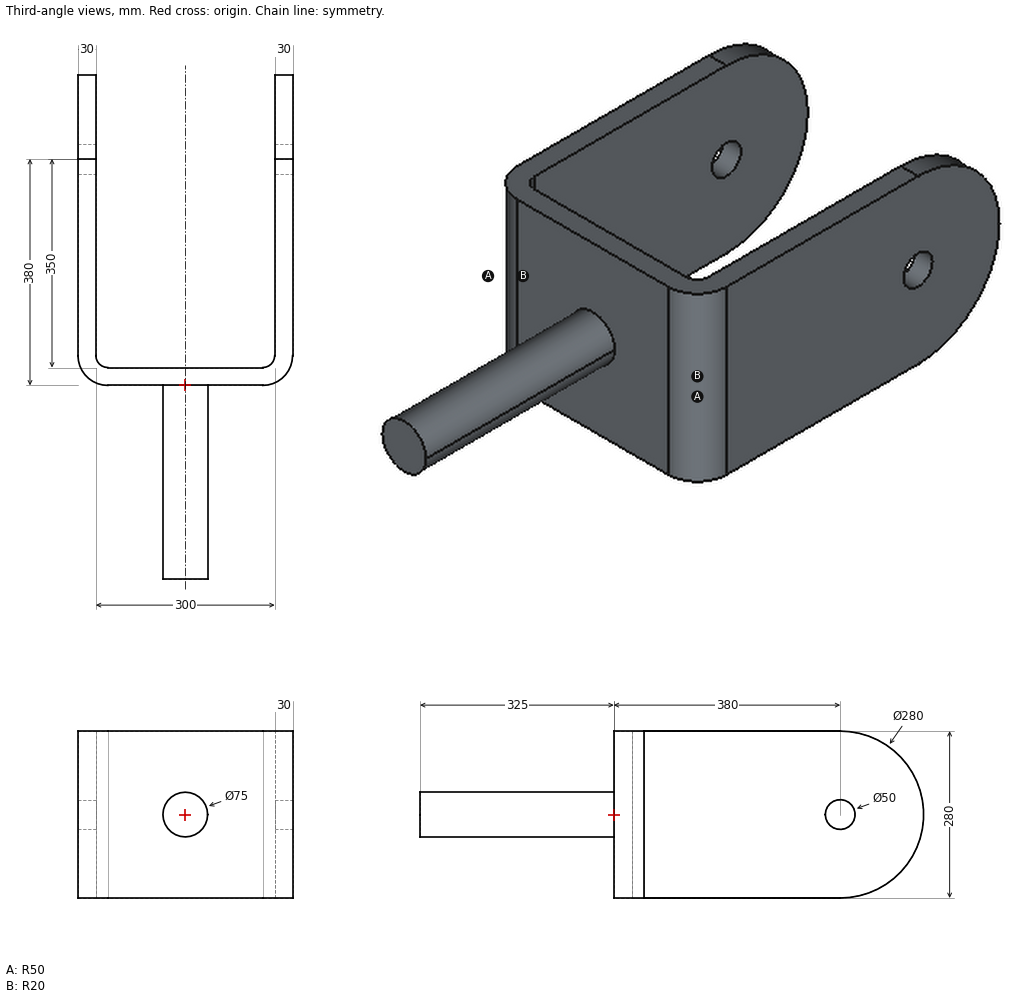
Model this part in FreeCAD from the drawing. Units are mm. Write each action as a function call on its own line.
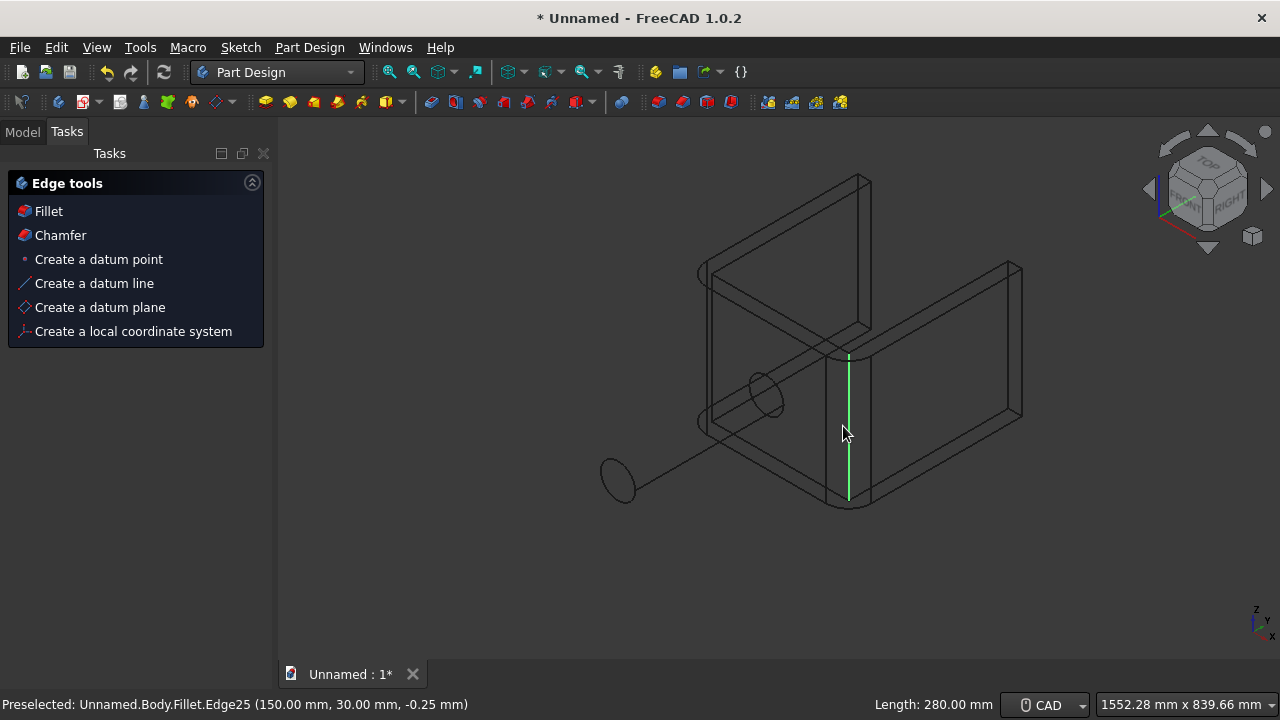
key(2)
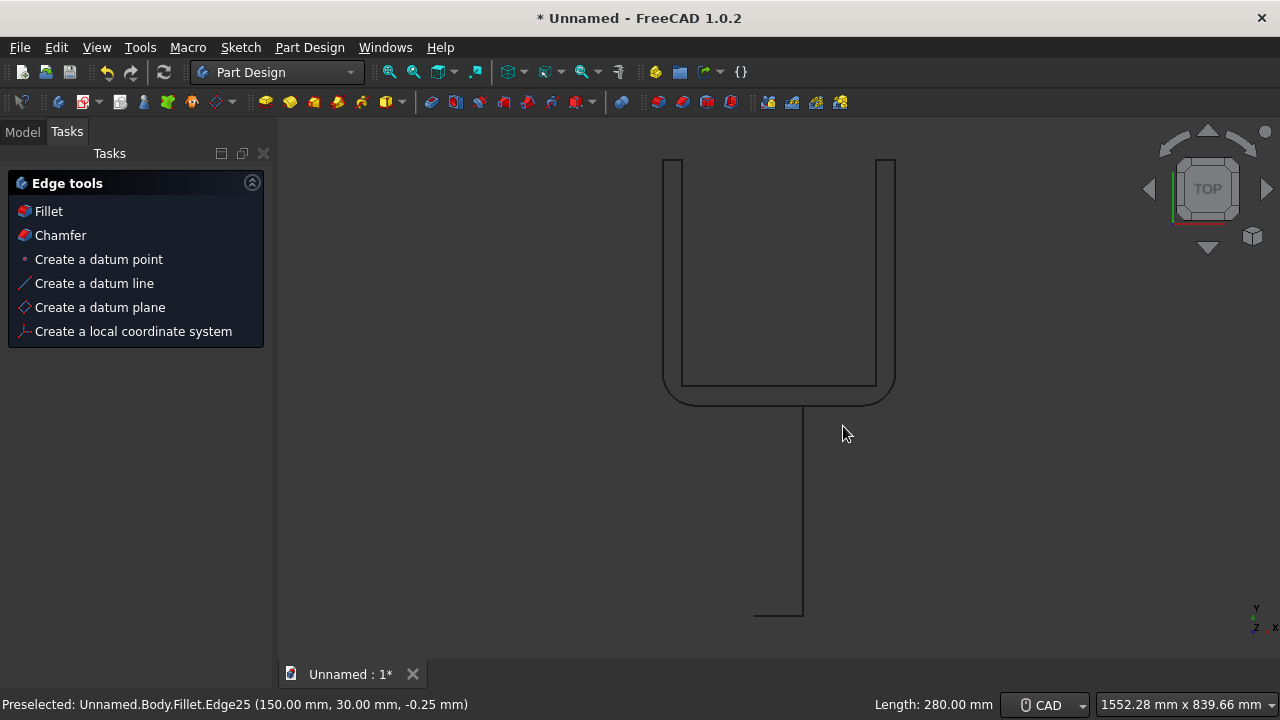
key(1)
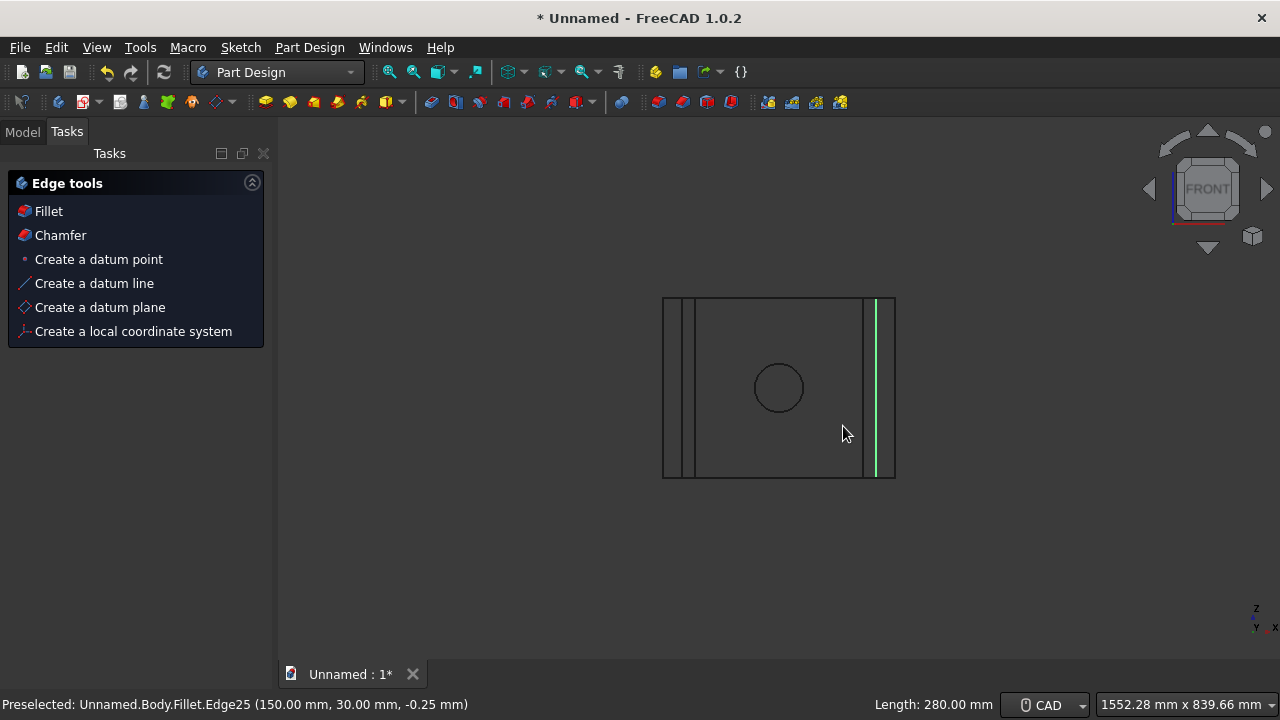
click(390, 72)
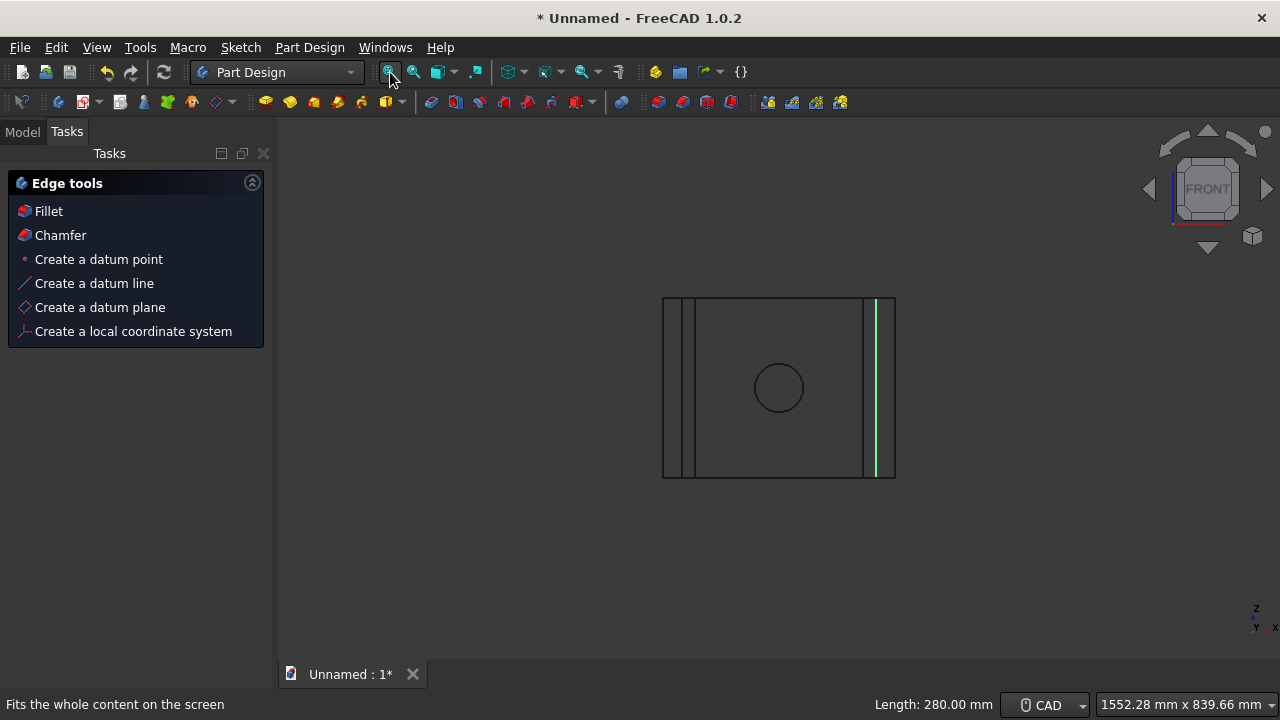
click(682, 387, ctrl)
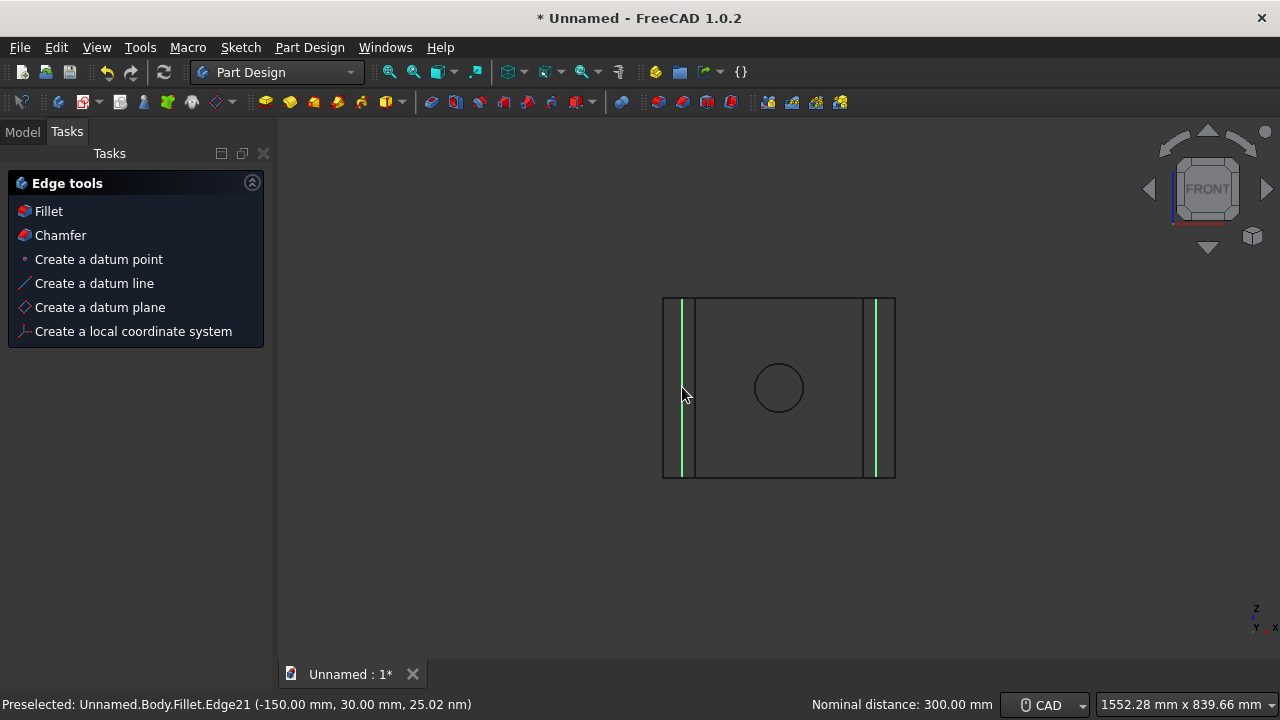
key(v)
key(1)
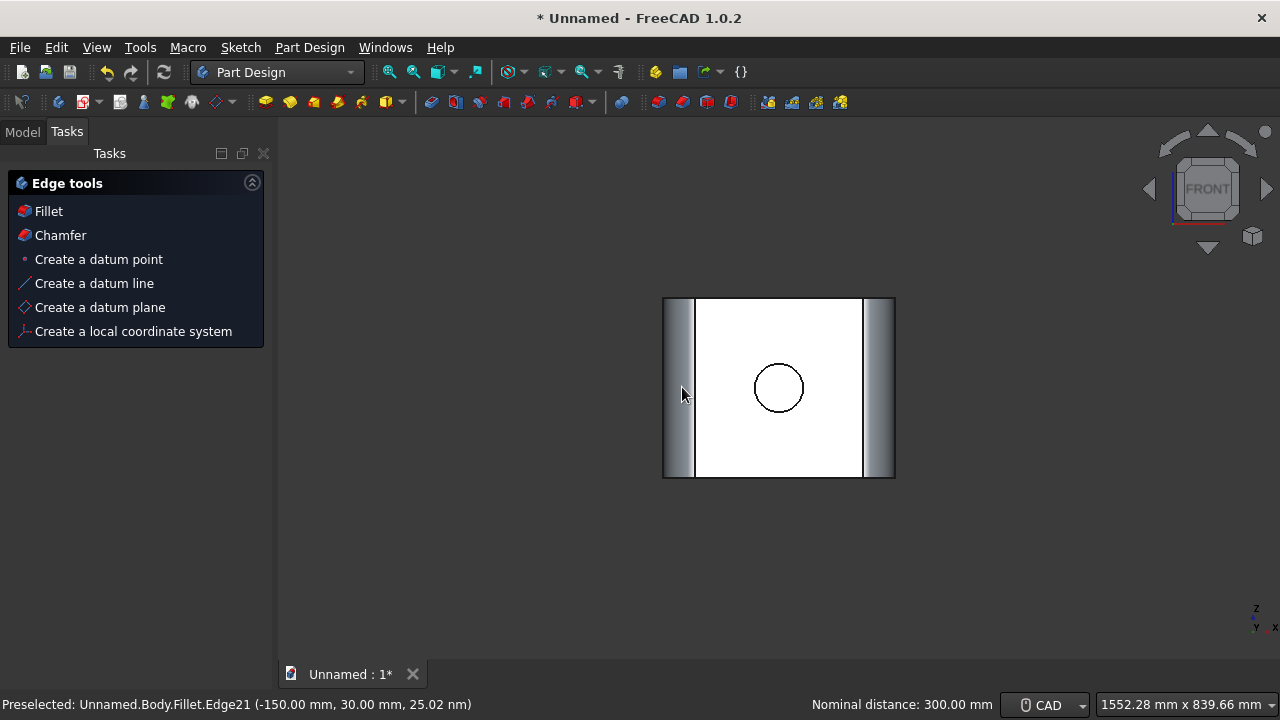
click(660, 102)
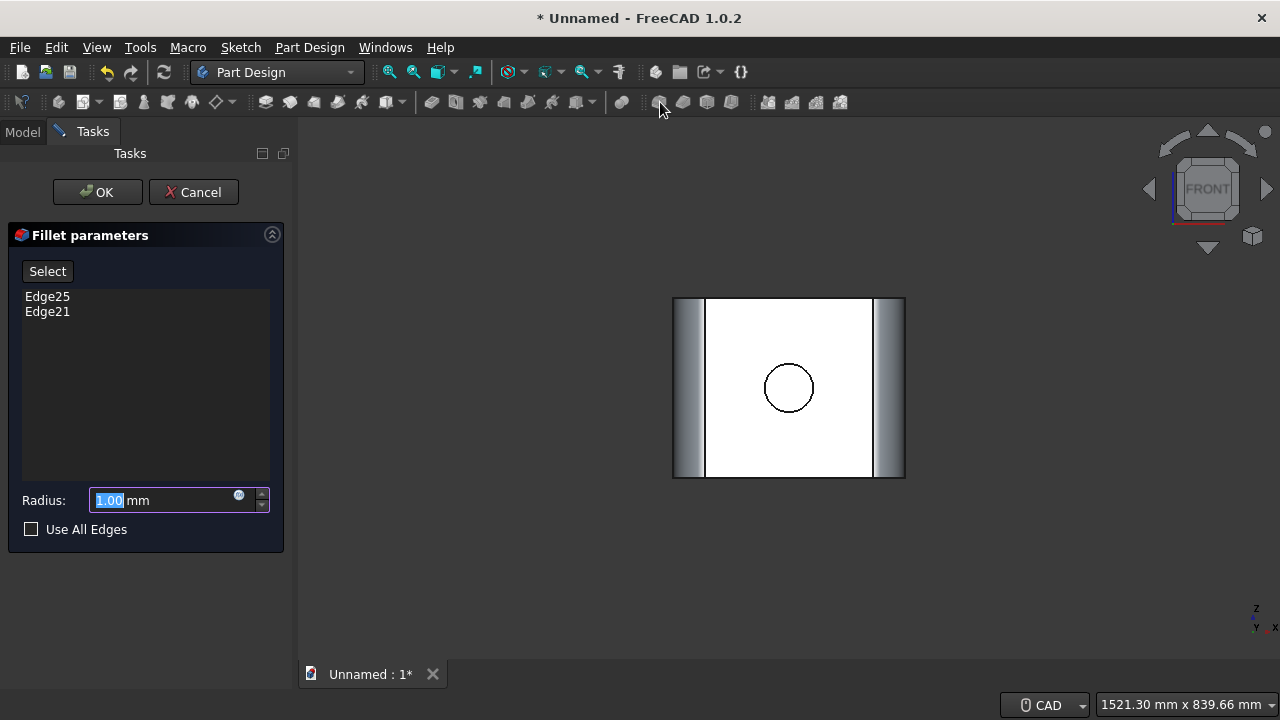
text(20)
key(Tab)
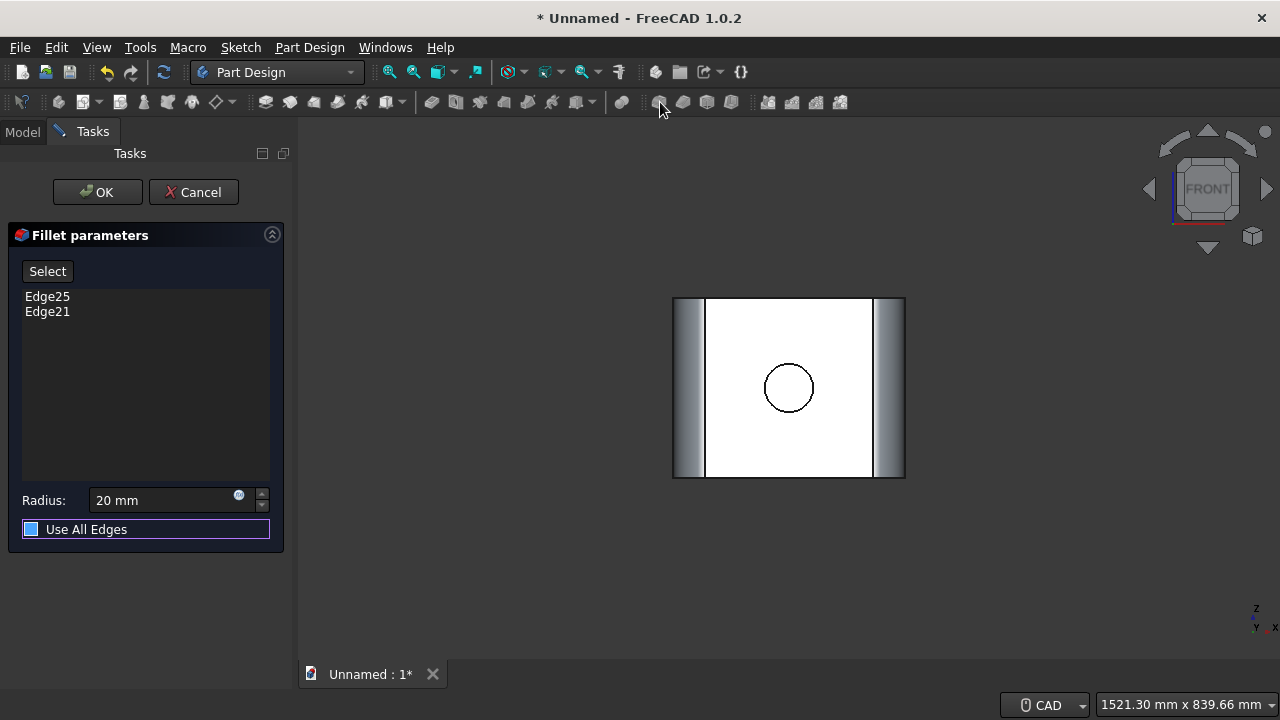
click(98, 192)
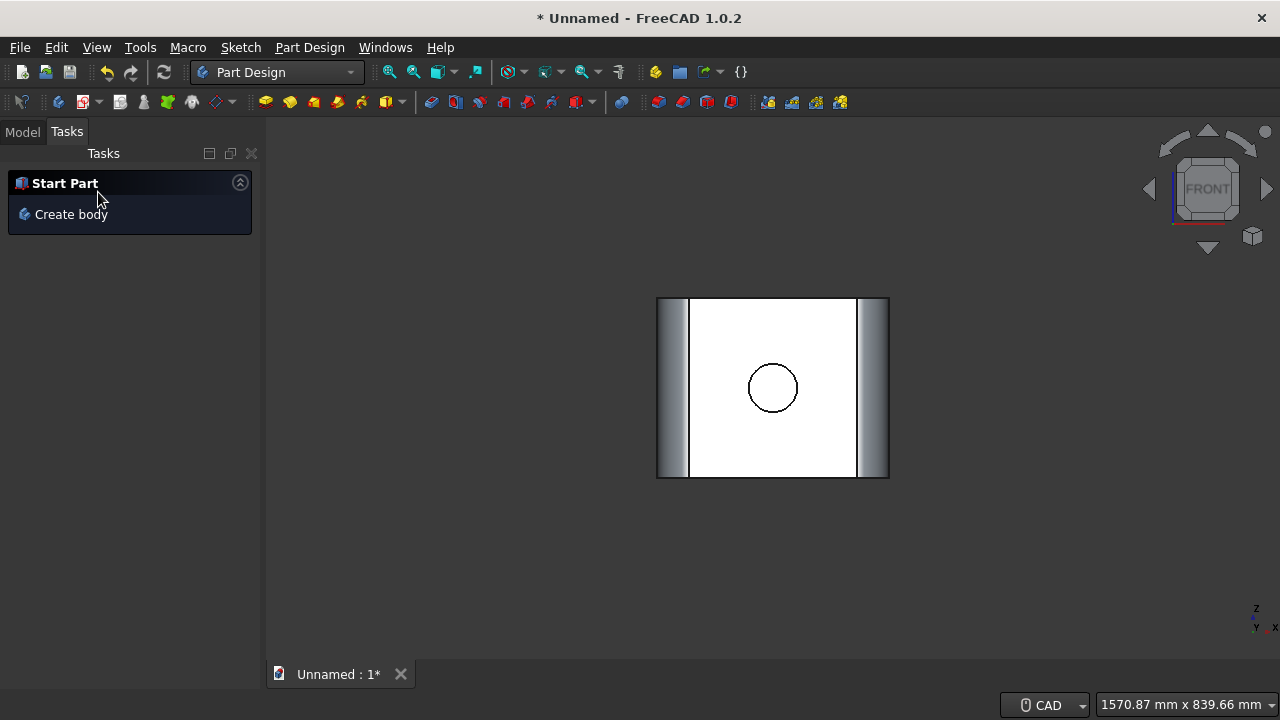
click(390, 72)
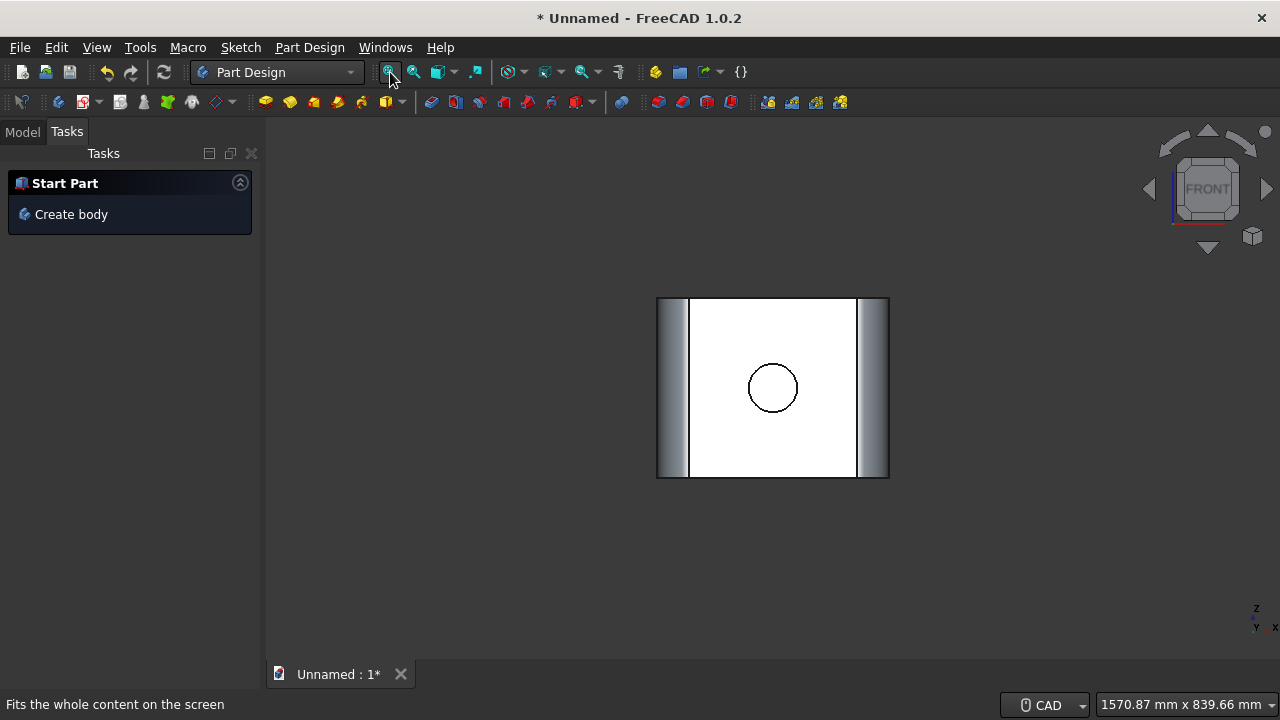
key(0)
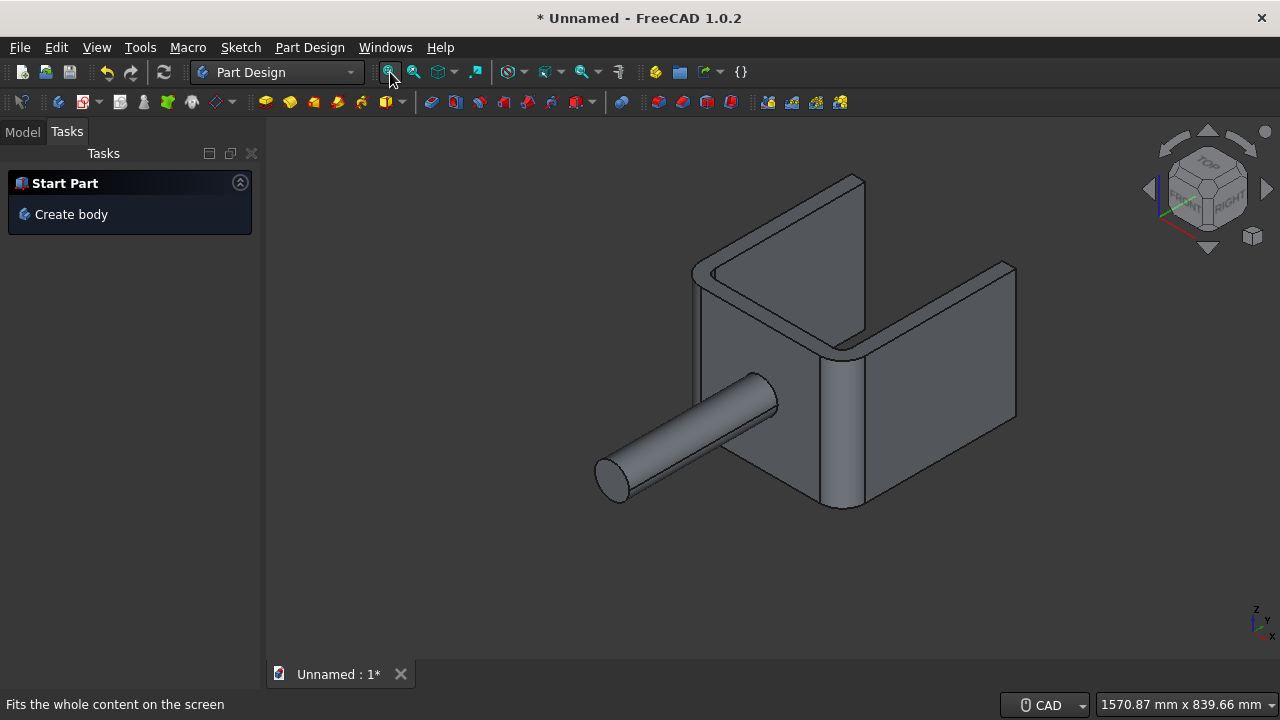
click(941, 385)